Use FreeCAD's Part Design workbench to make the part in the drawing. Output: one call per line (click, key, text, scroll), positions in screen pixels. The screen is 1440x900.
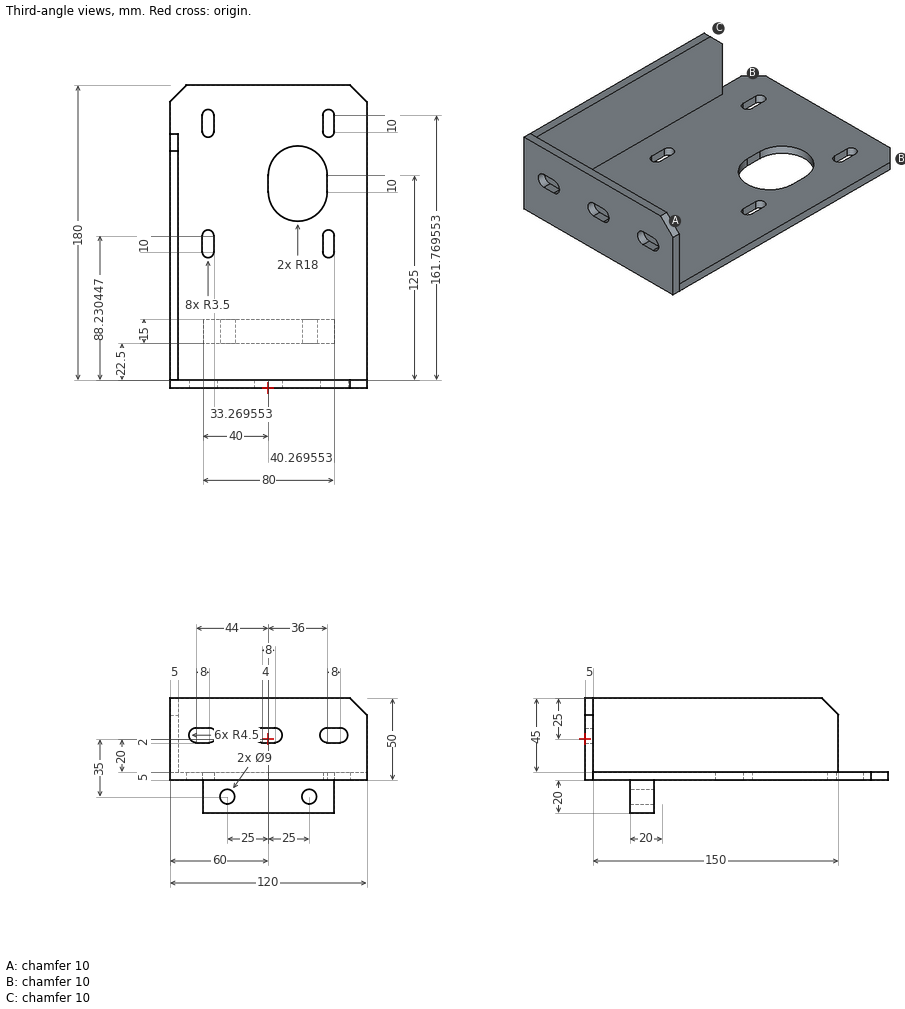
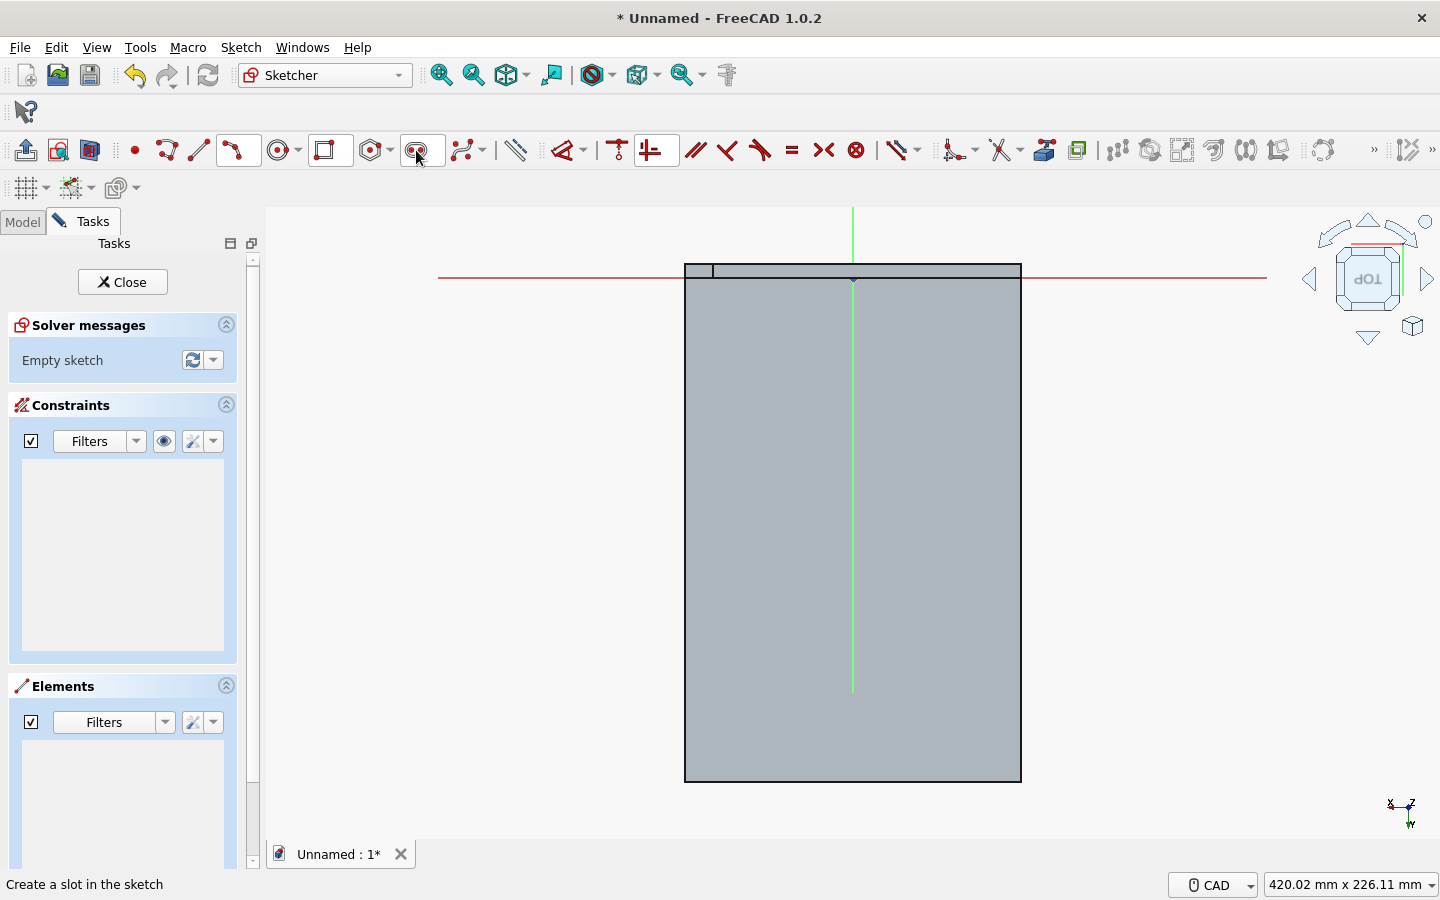
scroll(956, 525, up, 5)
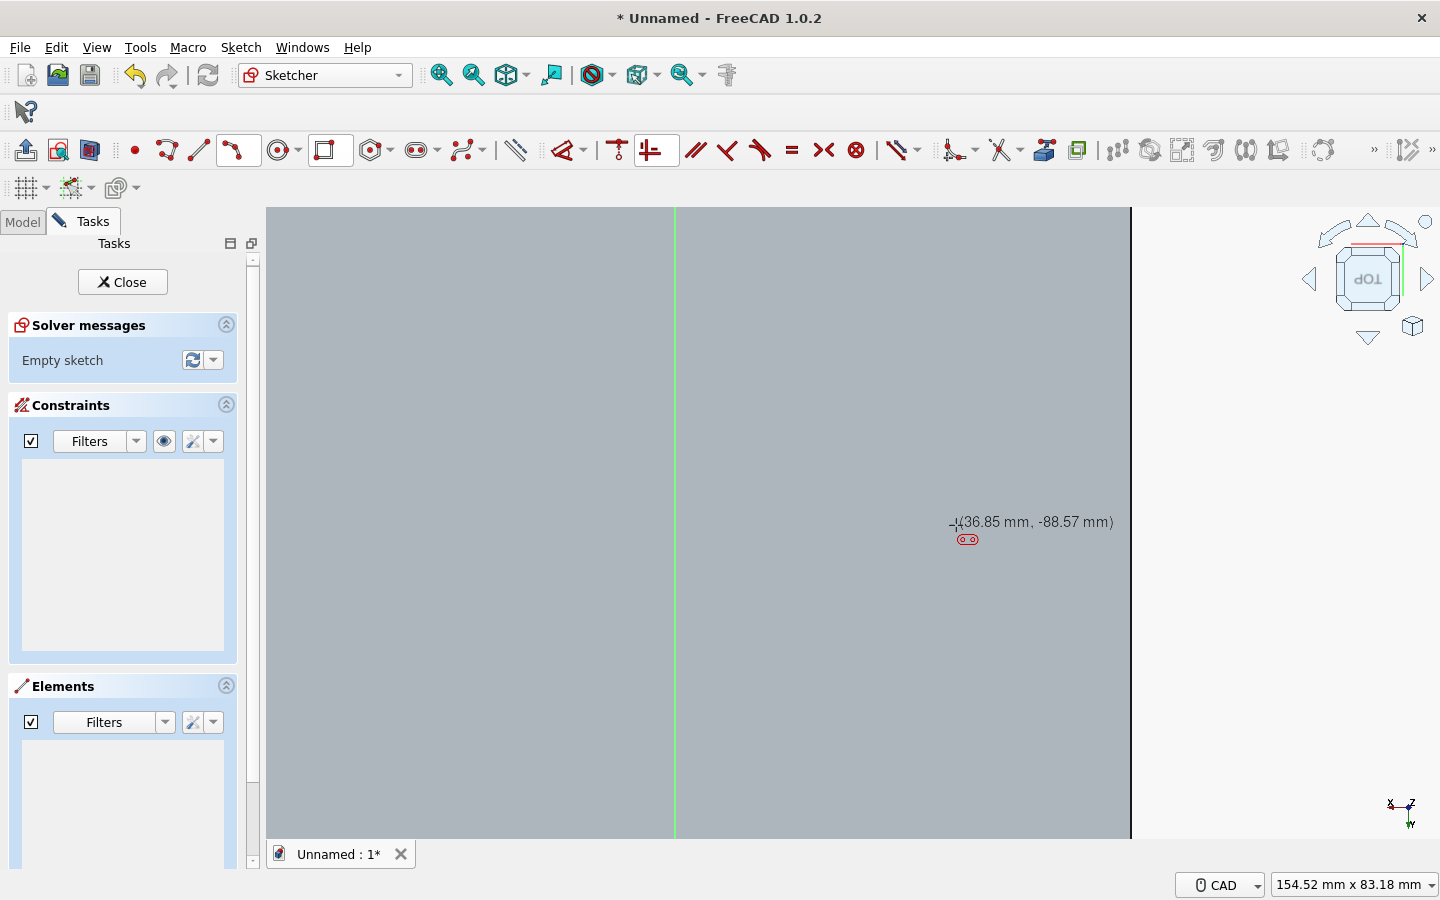
click(954, 524)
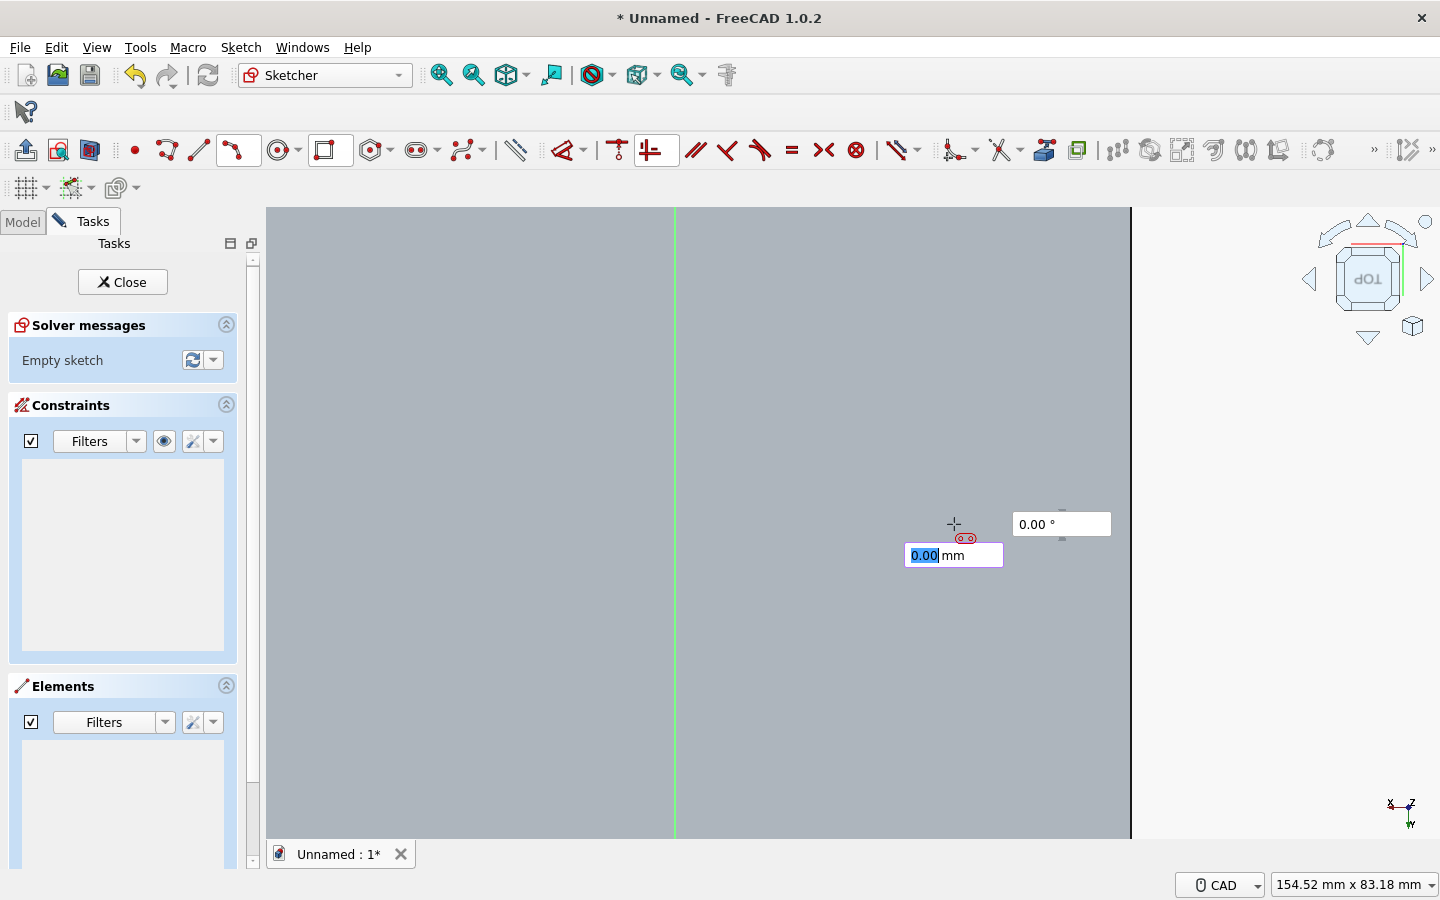
click(954, 448)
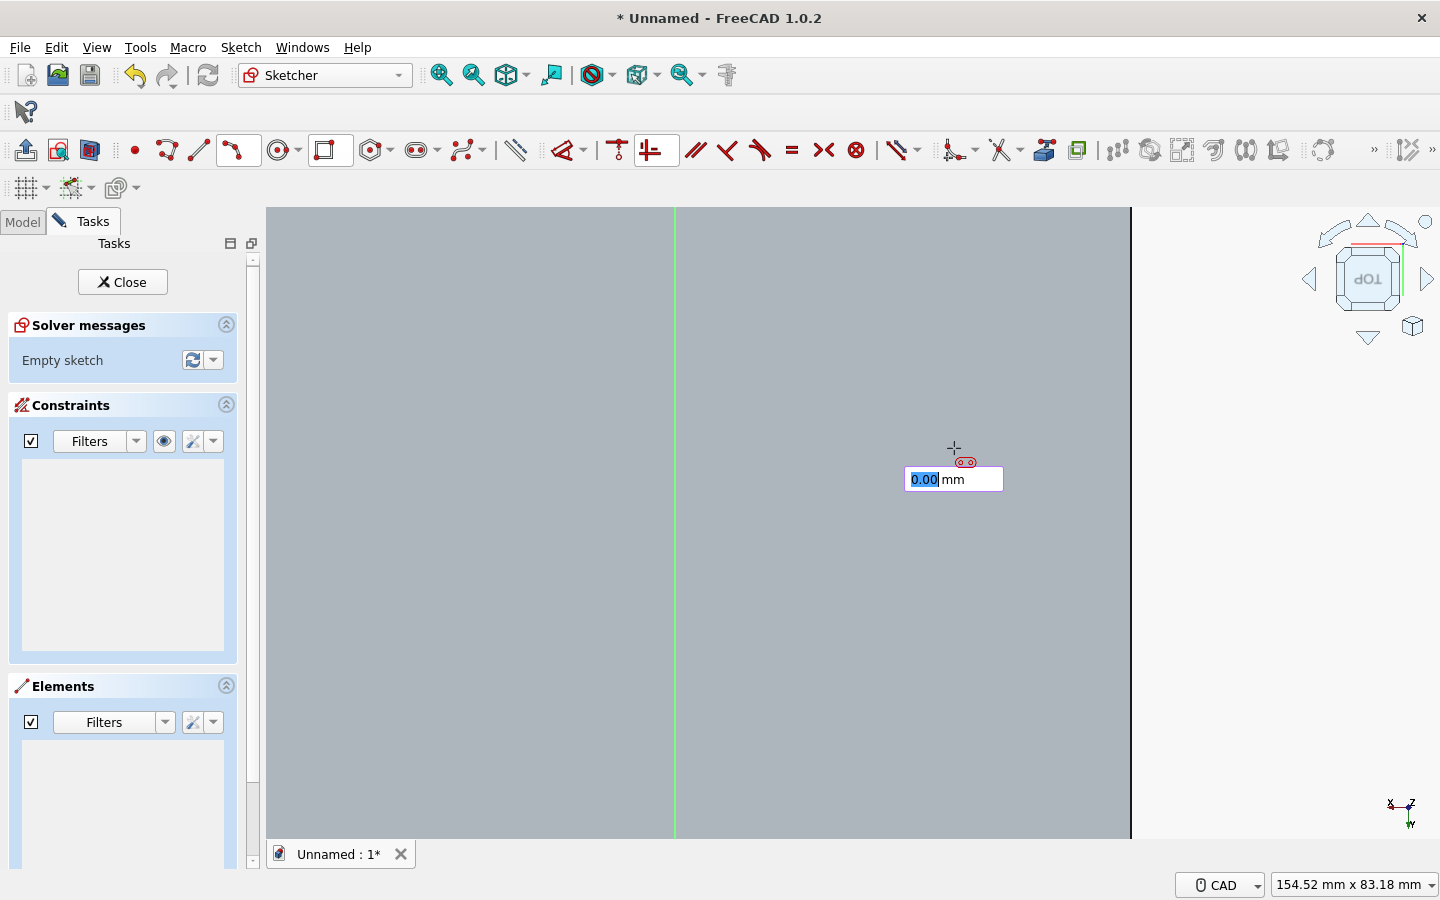
click(981, 486)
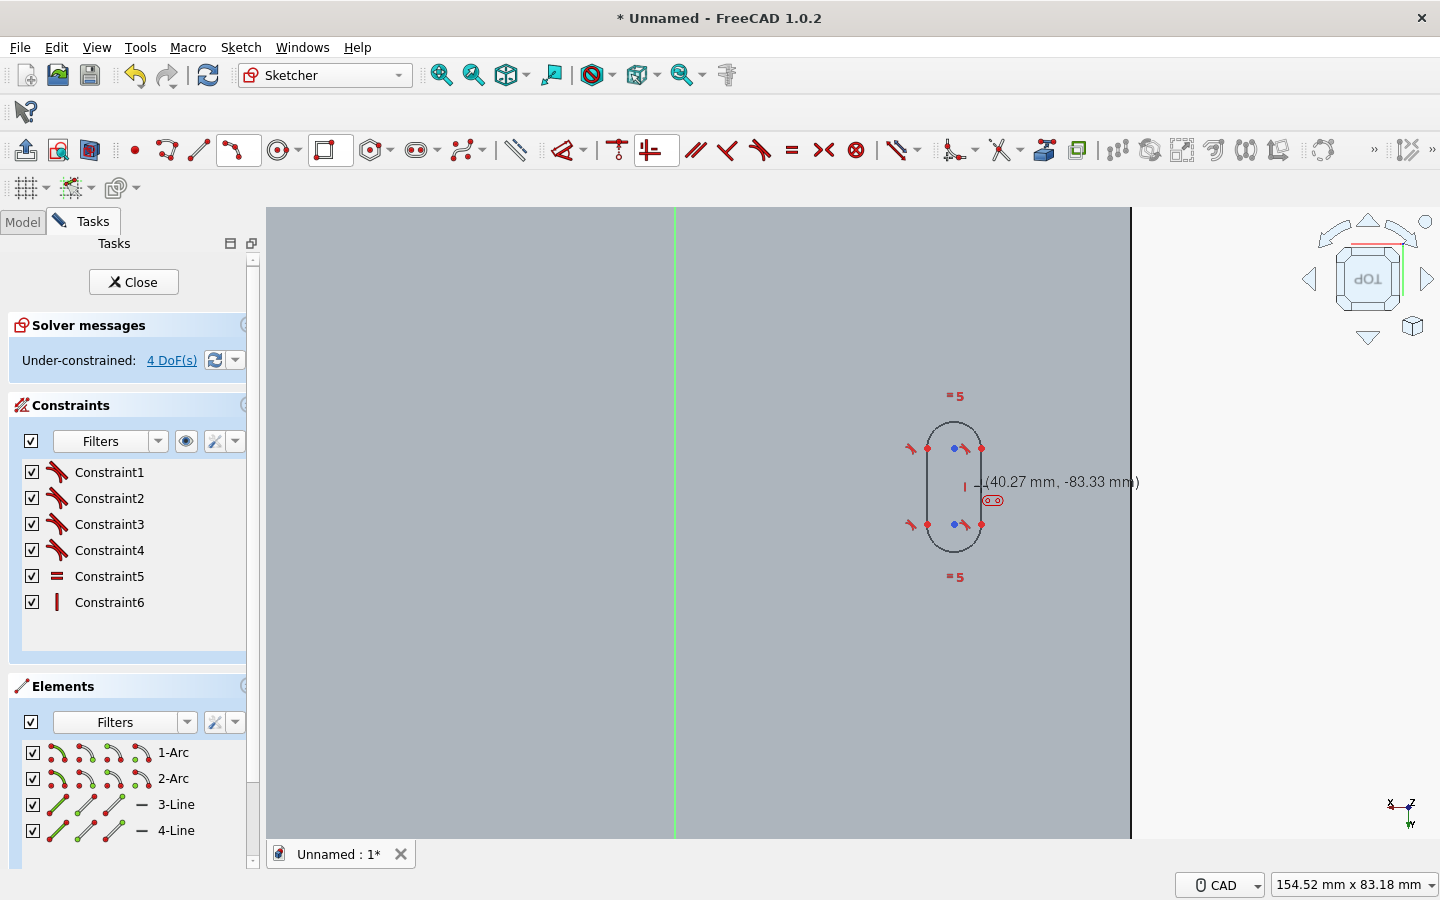
click(396, 524)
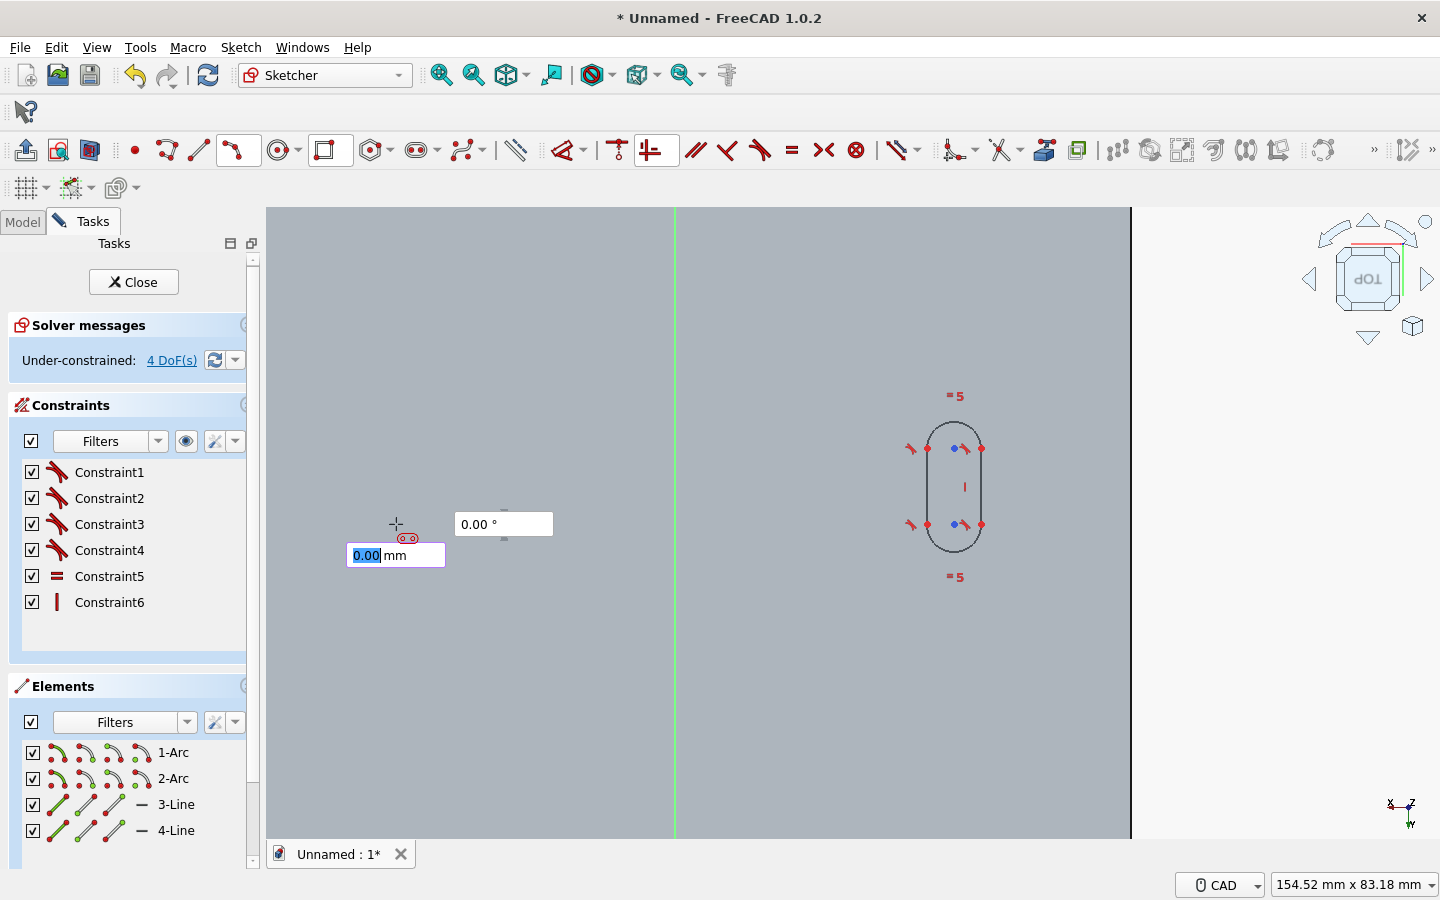
click(396, 448)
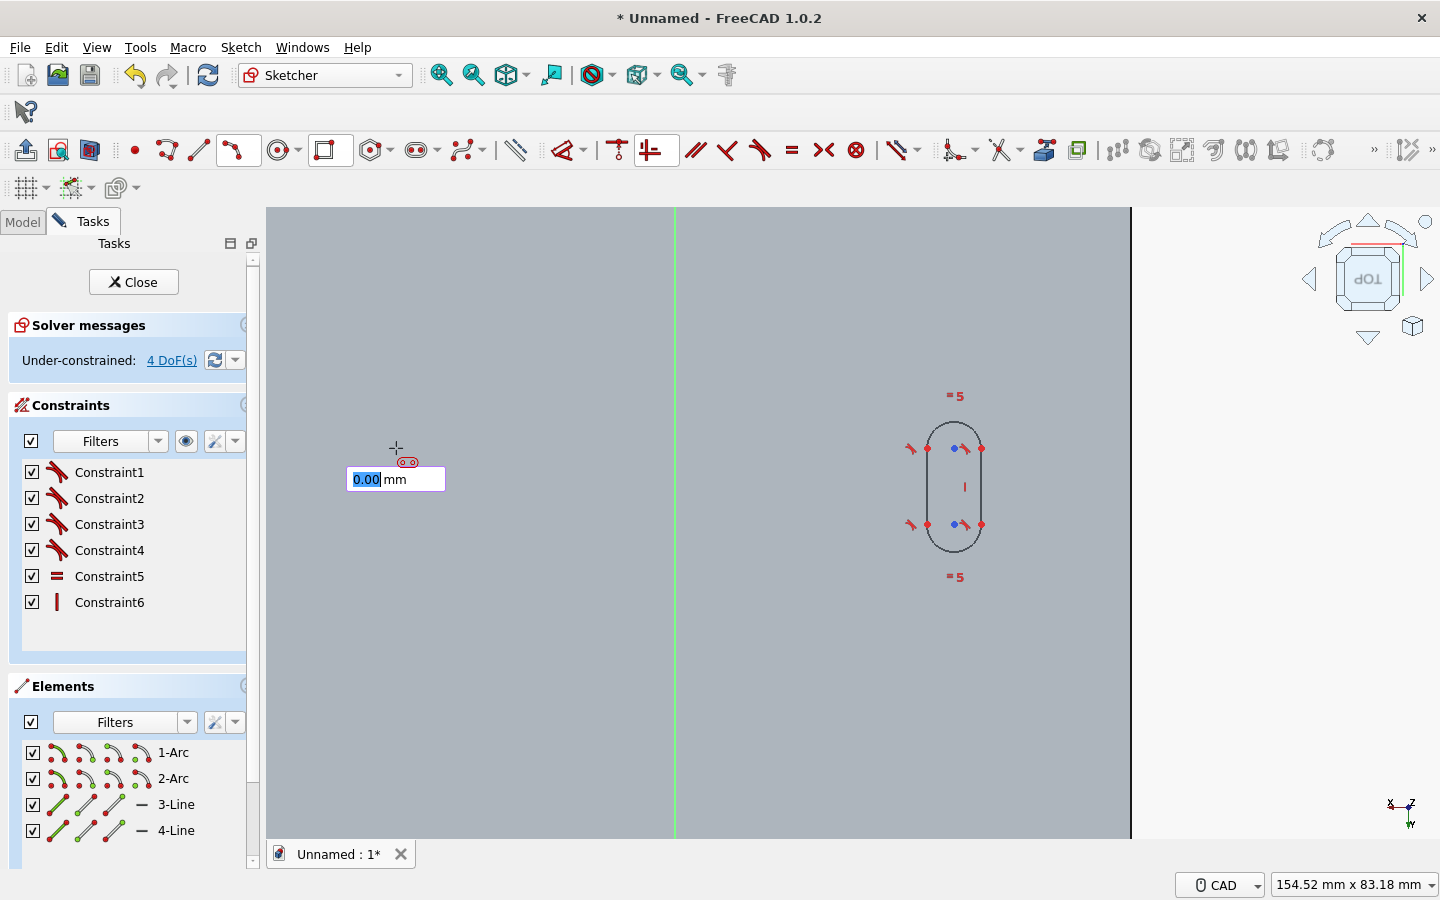
click(422, 486)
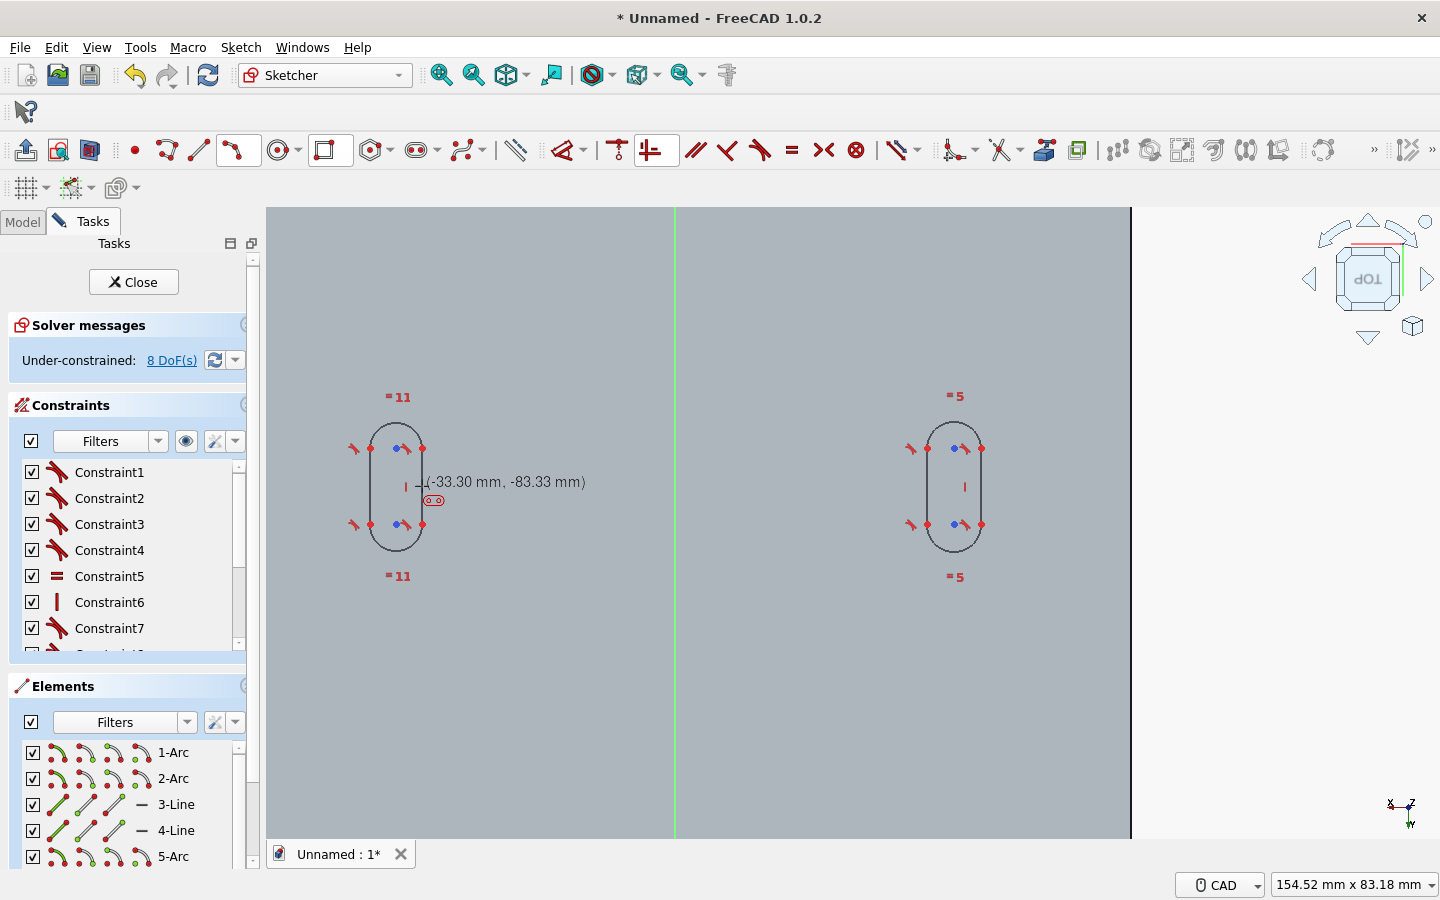
scroll(832, 541, down, 6)